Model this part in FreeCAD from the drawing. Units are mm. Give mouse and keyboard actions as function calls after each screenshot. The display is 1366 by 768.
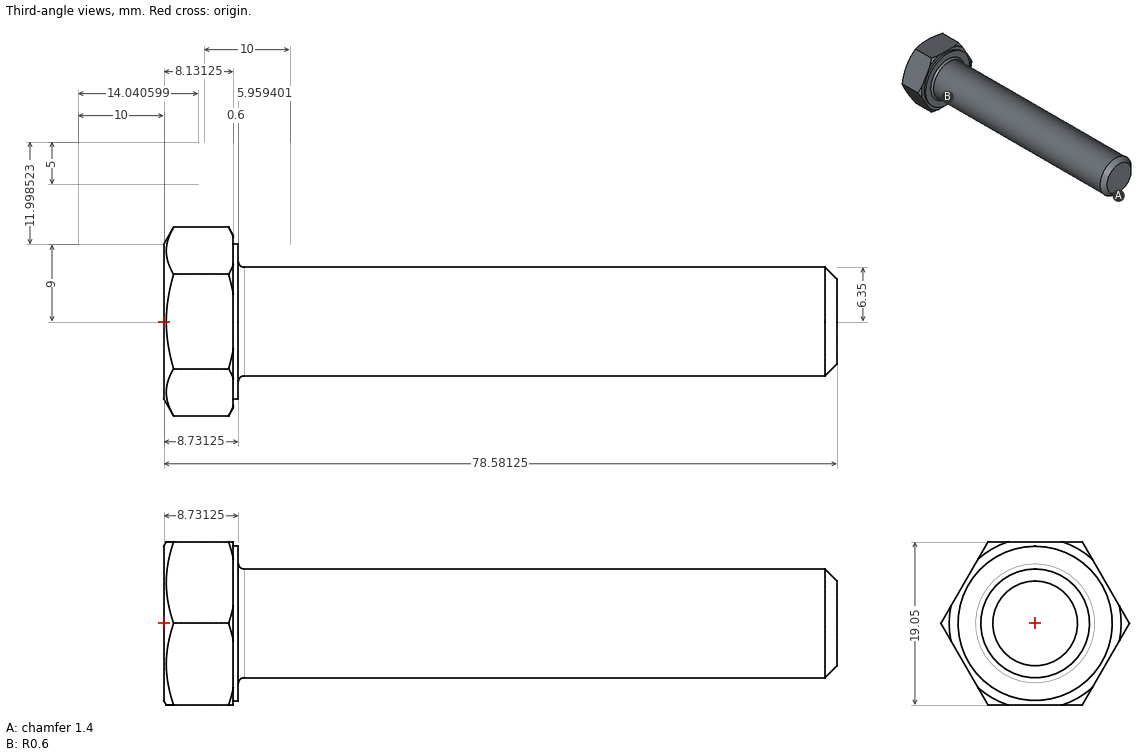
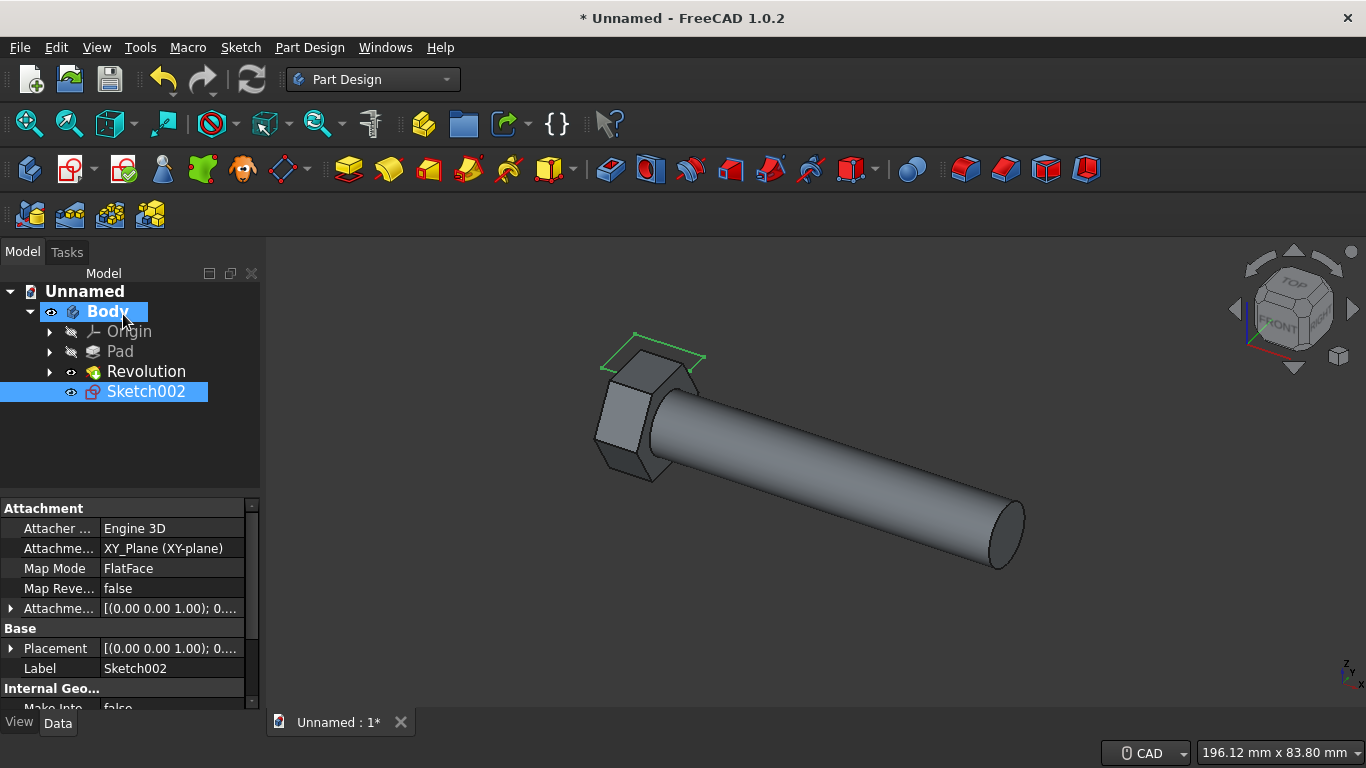
click(692, 170)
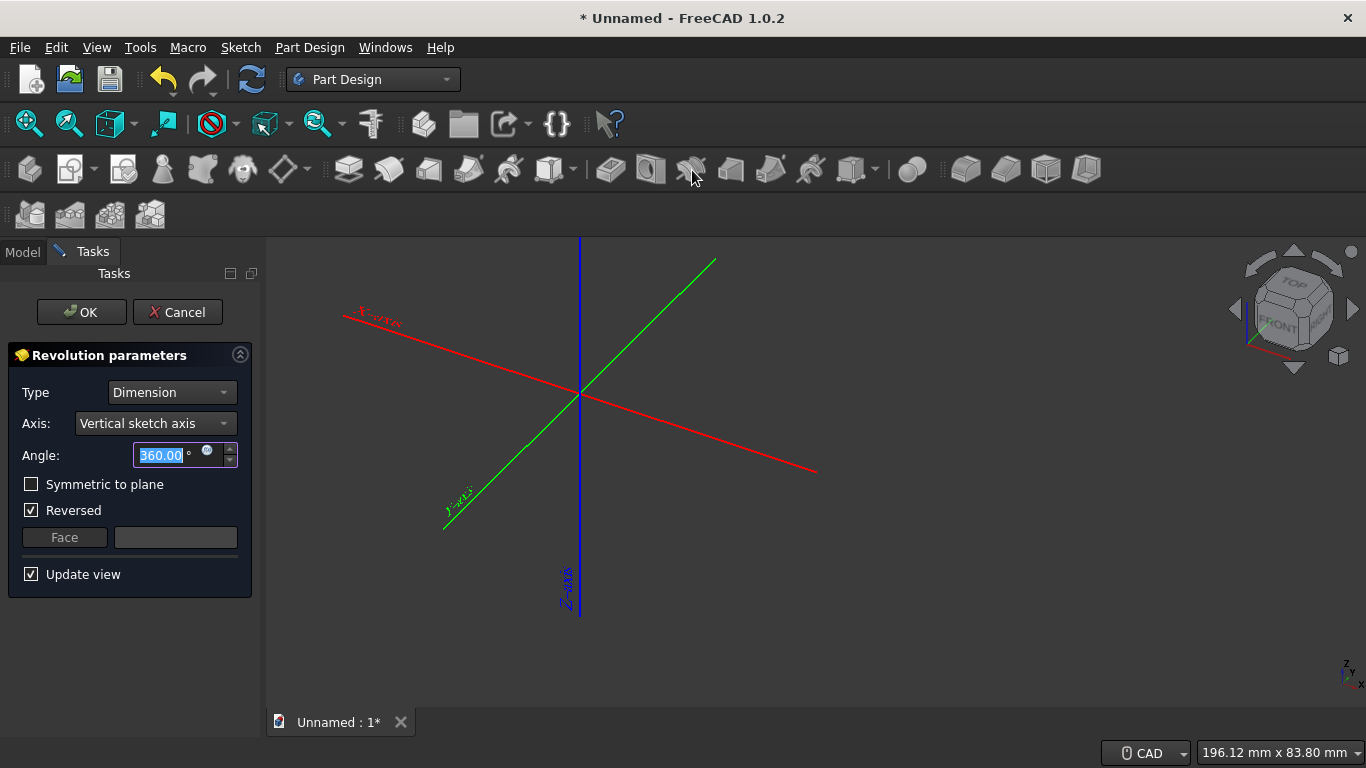
click(156, 424)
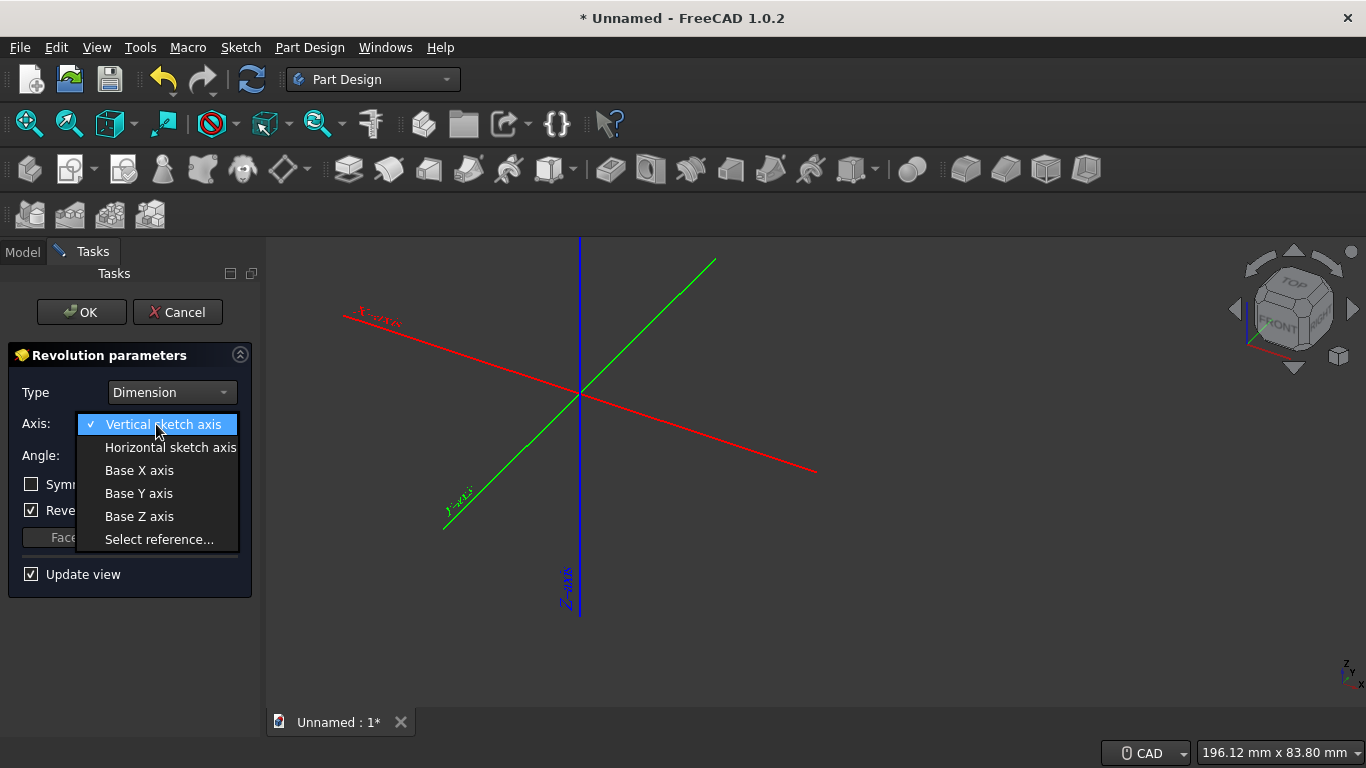
click(156, 448)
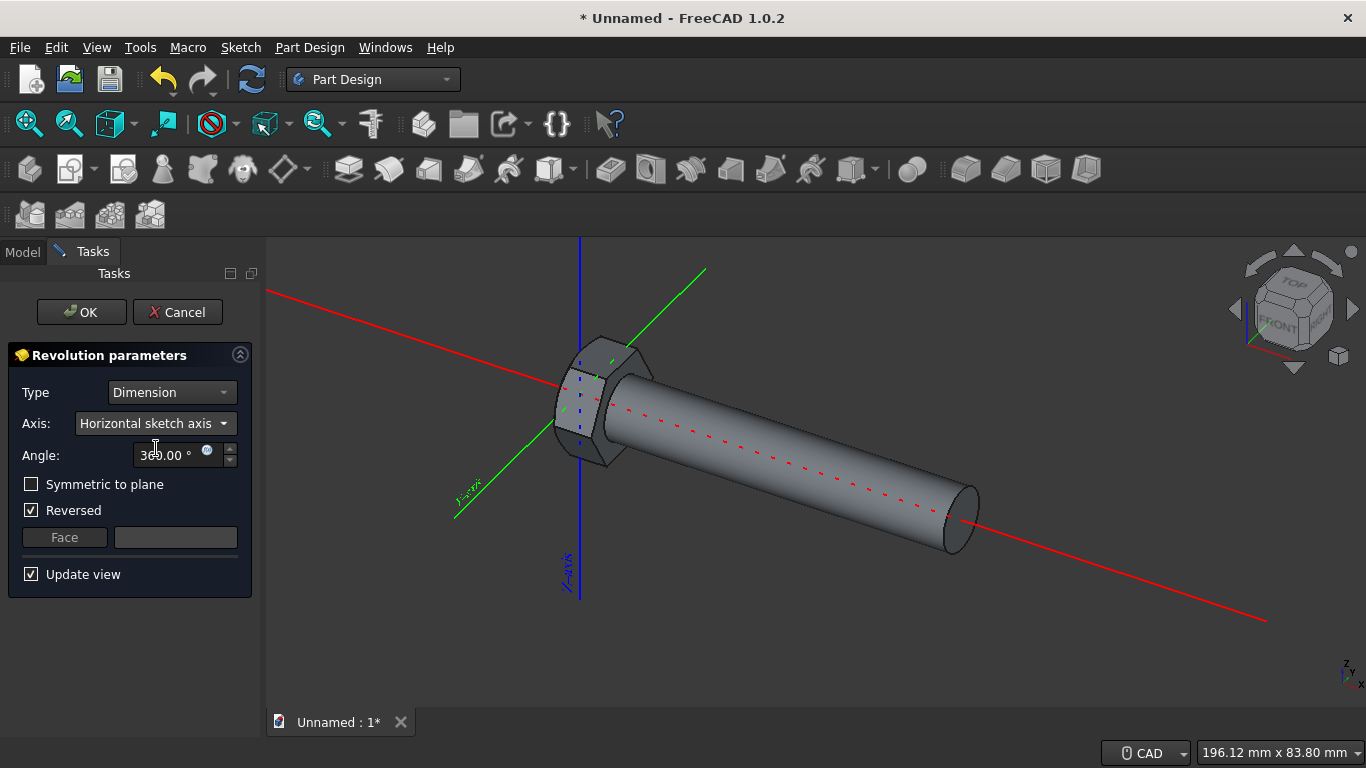
click(82, 312)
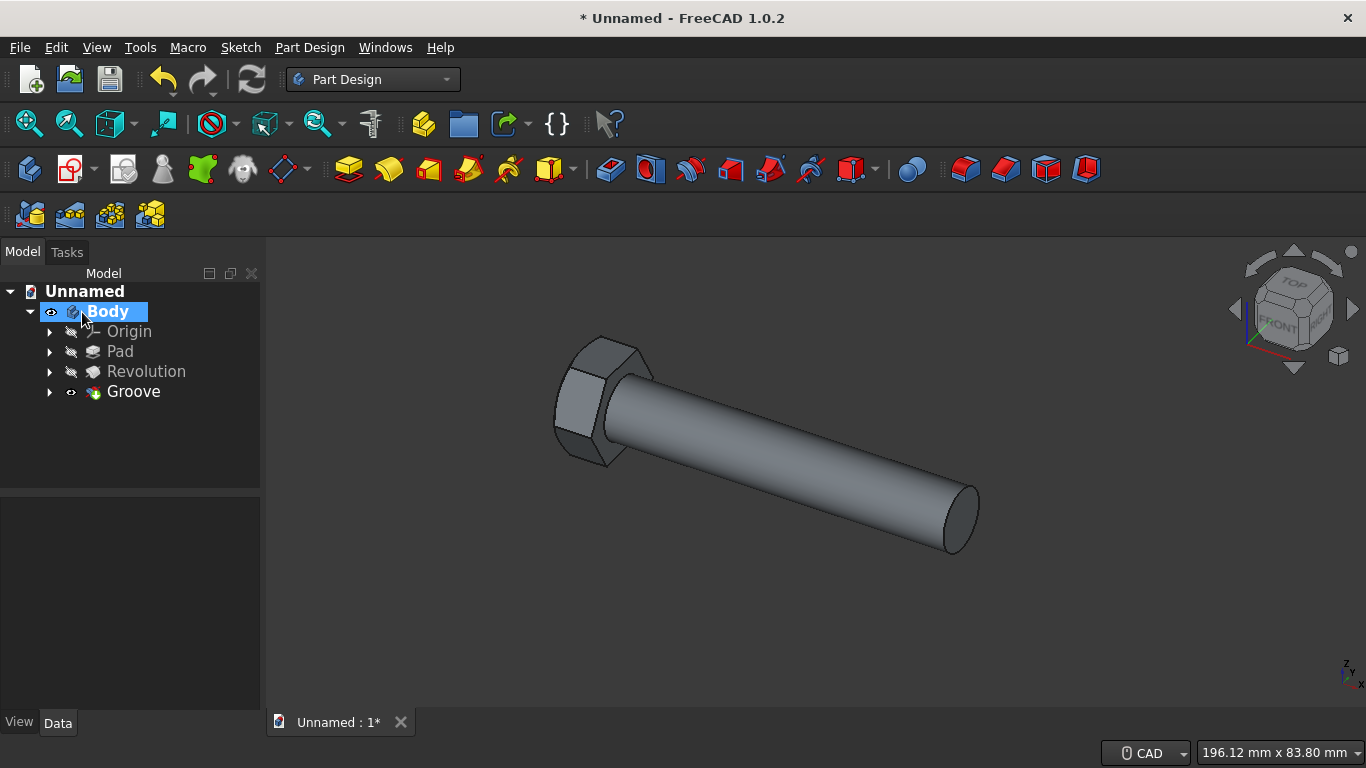
click(70, 170)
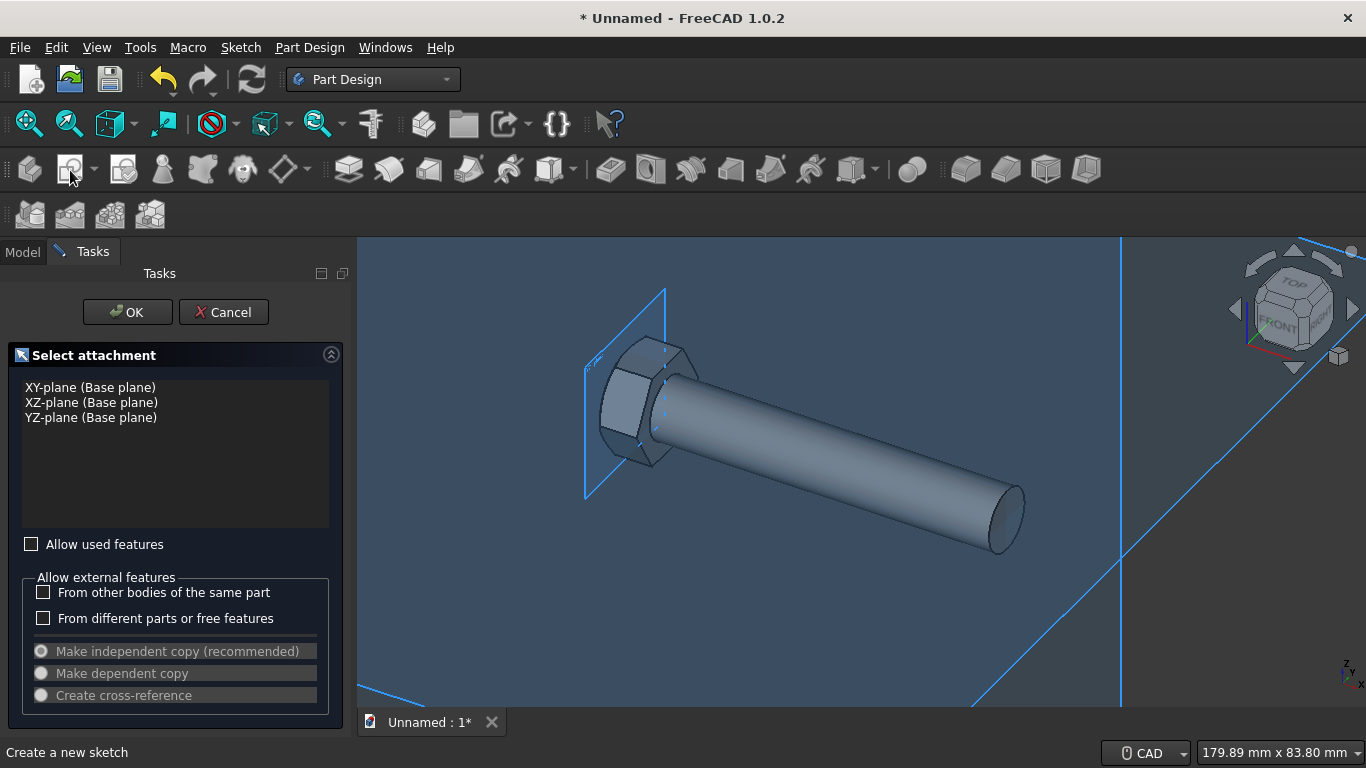
click(82, 388)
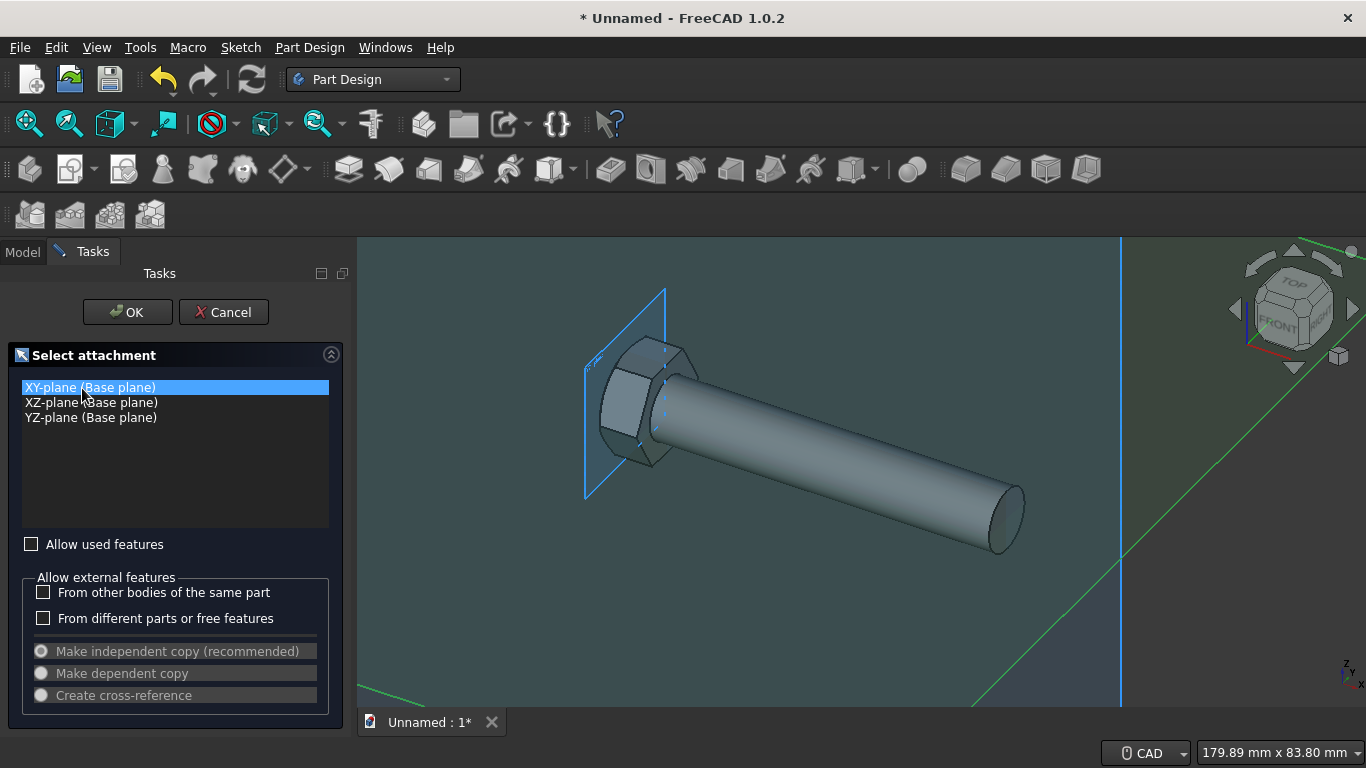
click(128, 312)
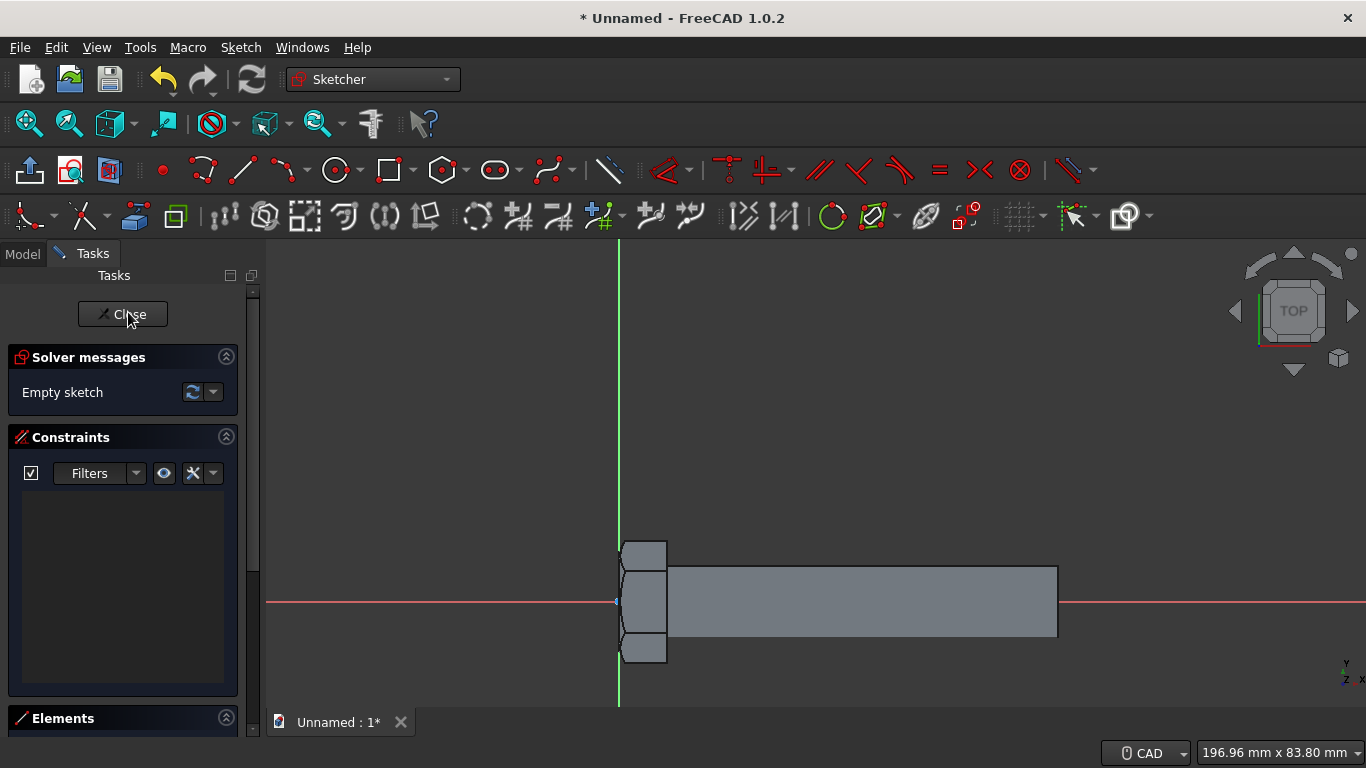
click(110, 170)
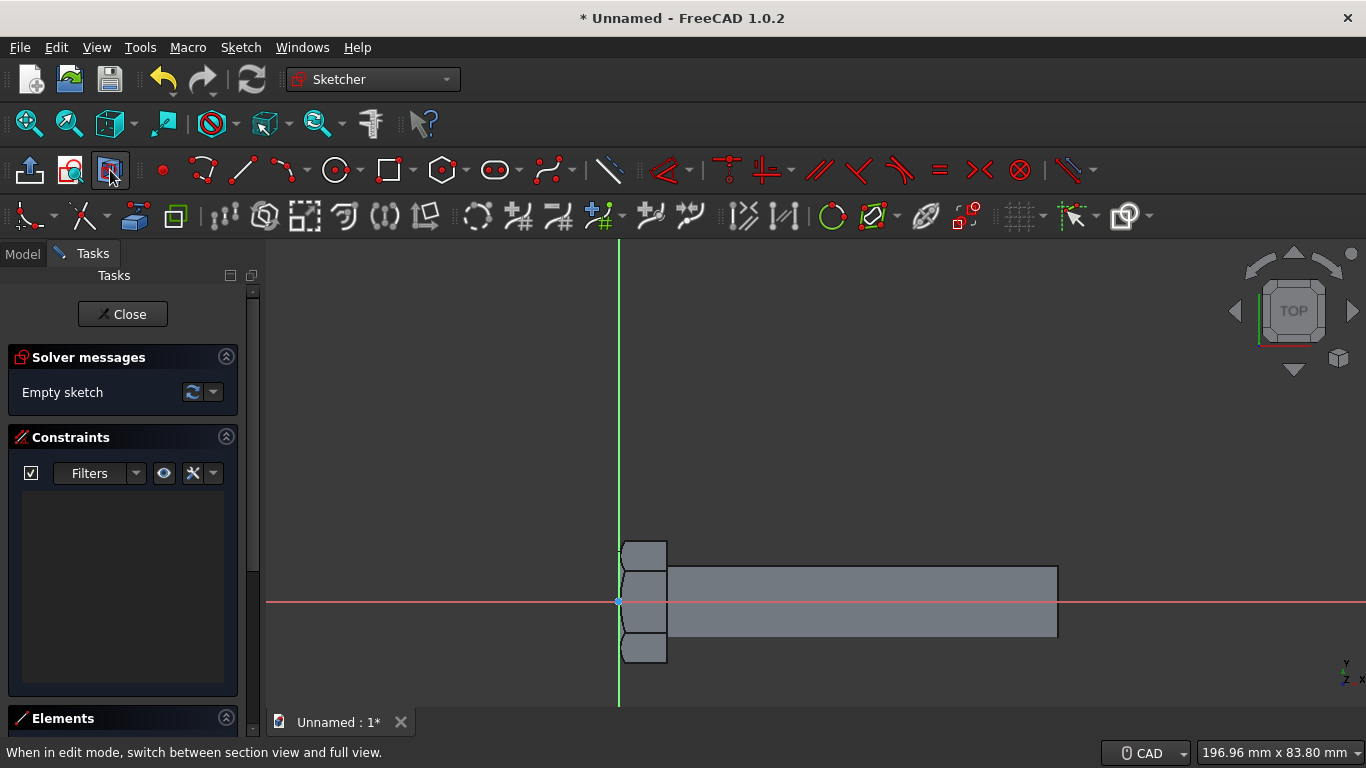
scroll(609, 584, up, 5)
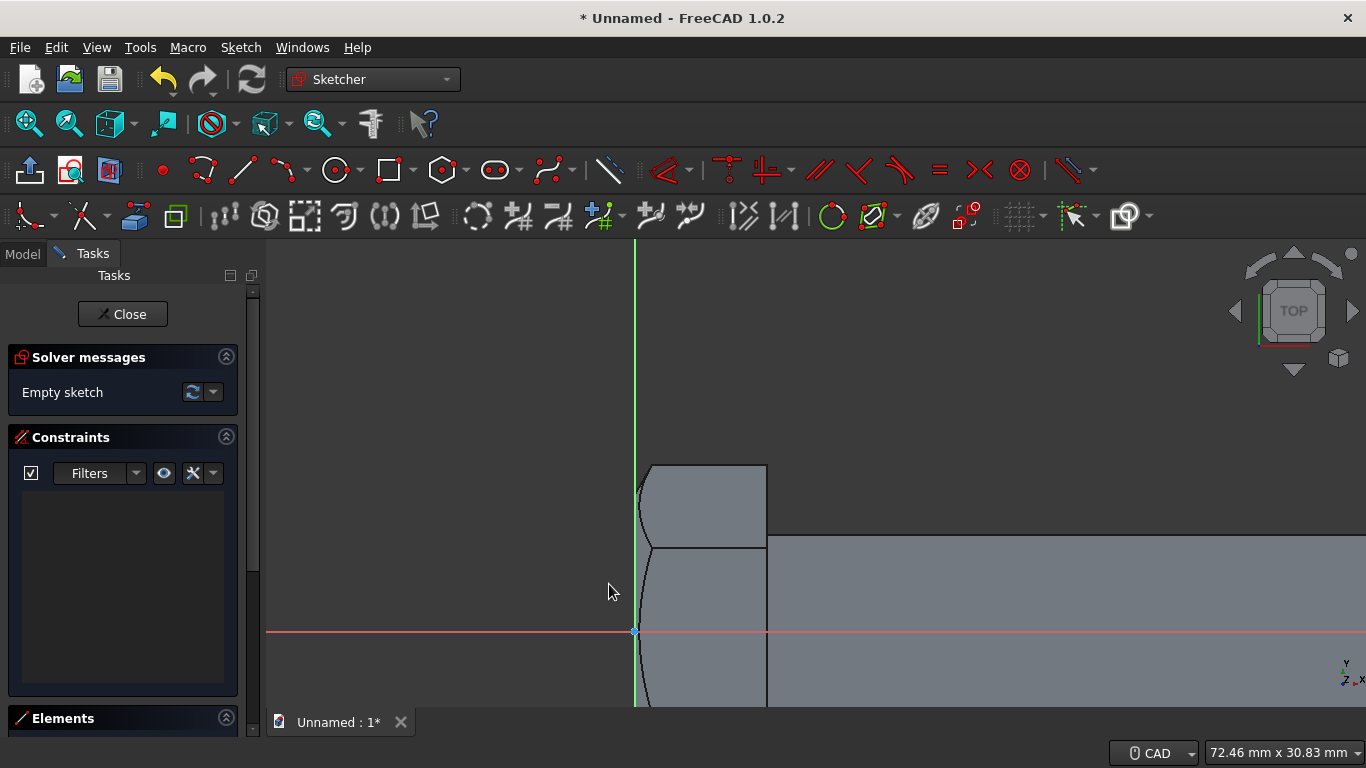
click(204, 170)